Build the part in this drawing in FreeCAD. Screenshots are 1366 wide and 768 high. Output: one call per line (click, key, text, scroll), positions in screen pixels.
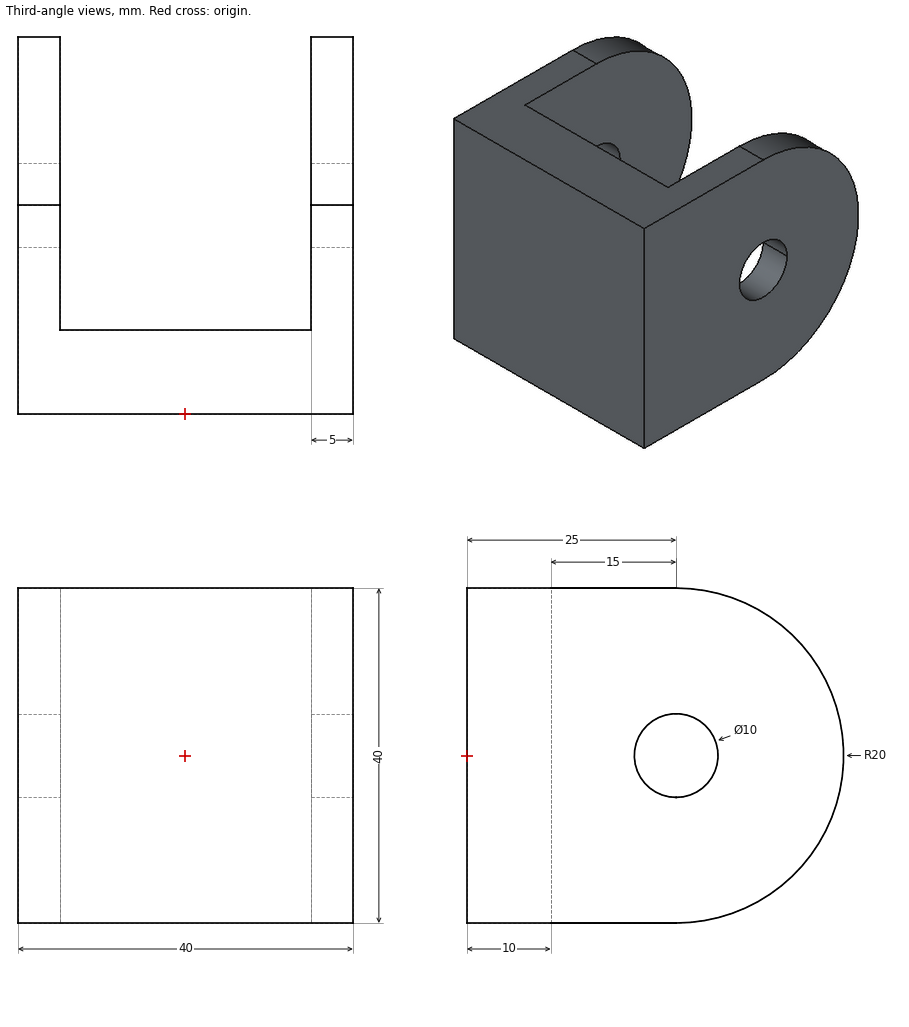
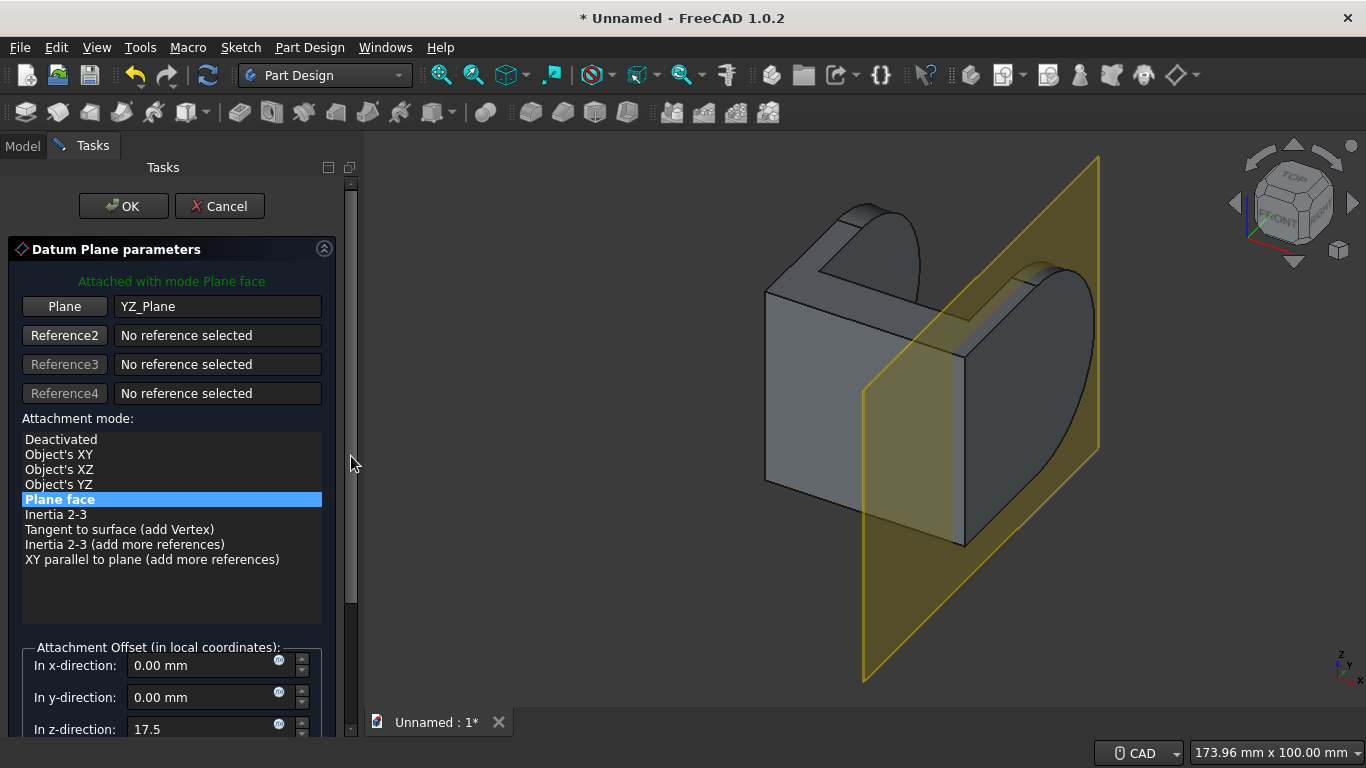
click(124, 206)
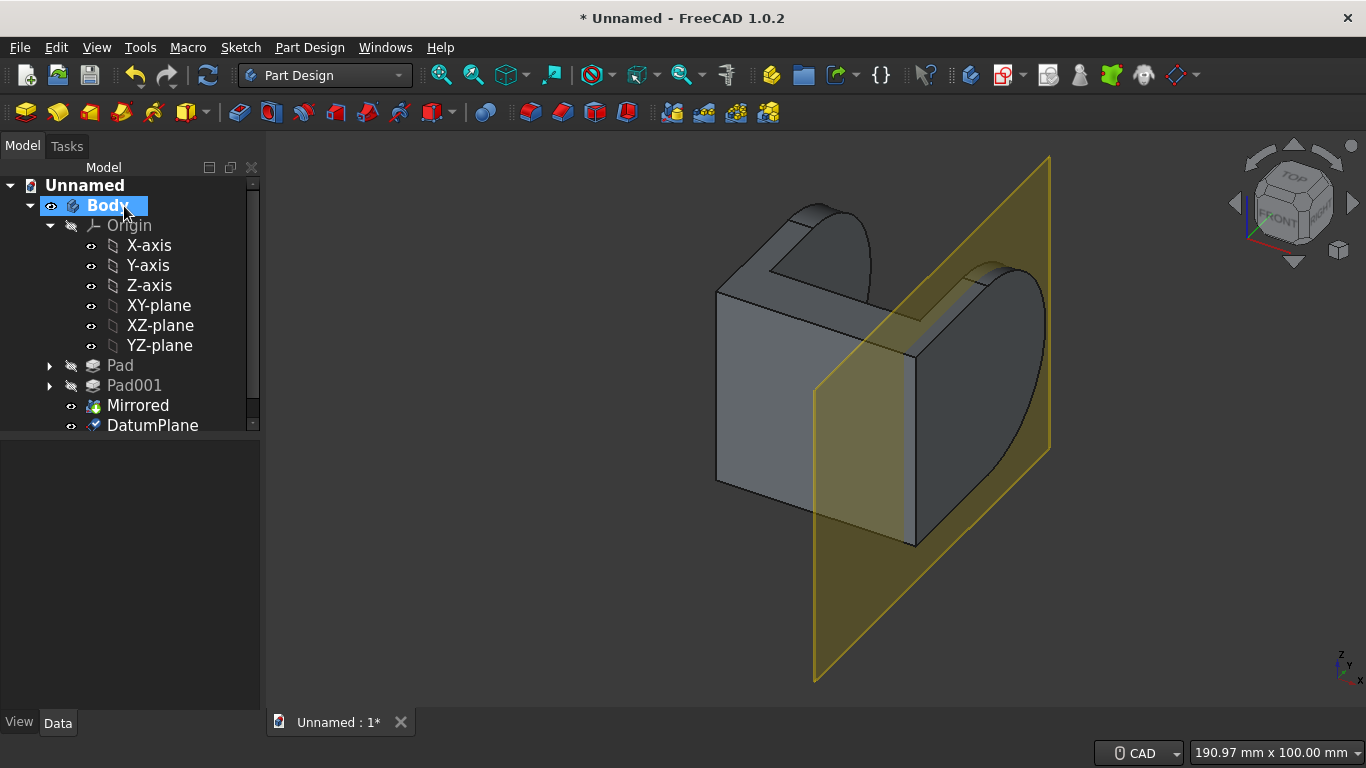
click(116, 426)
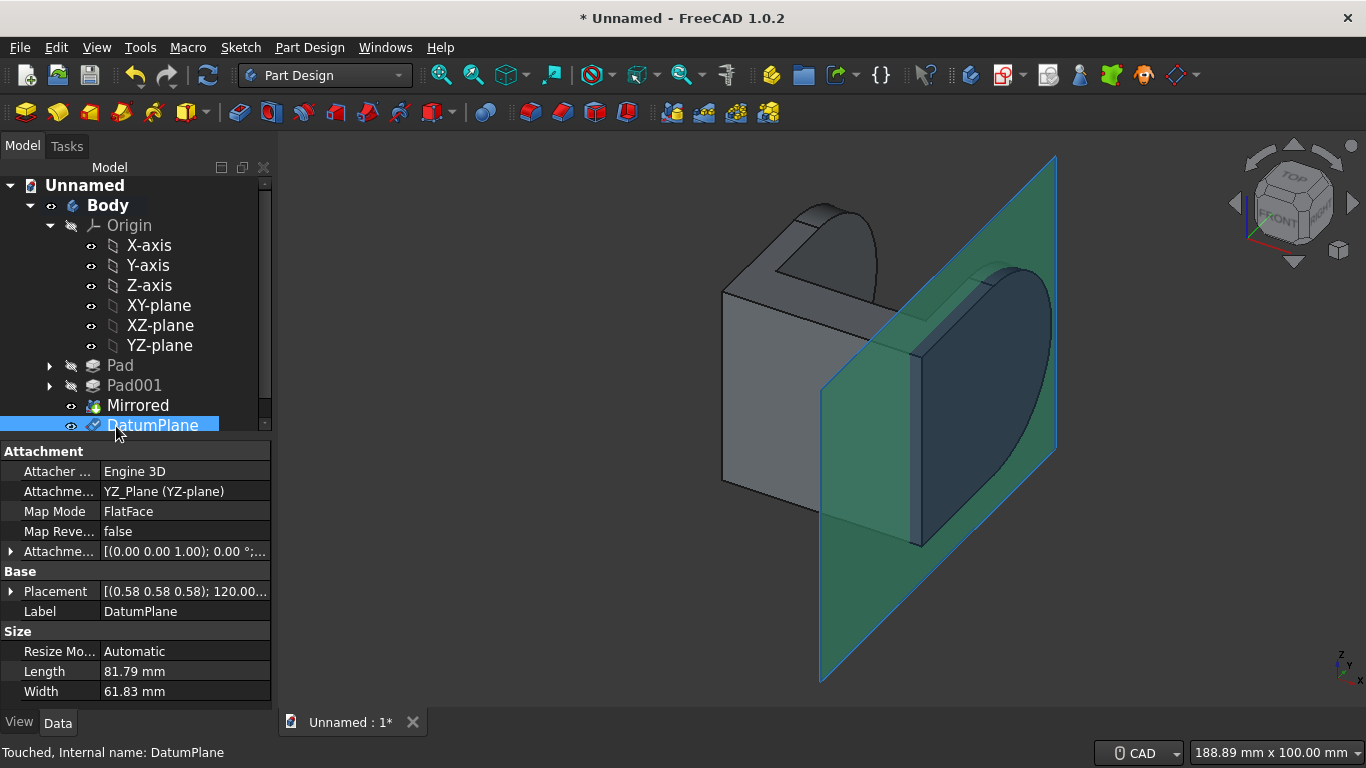
click(1004, 76)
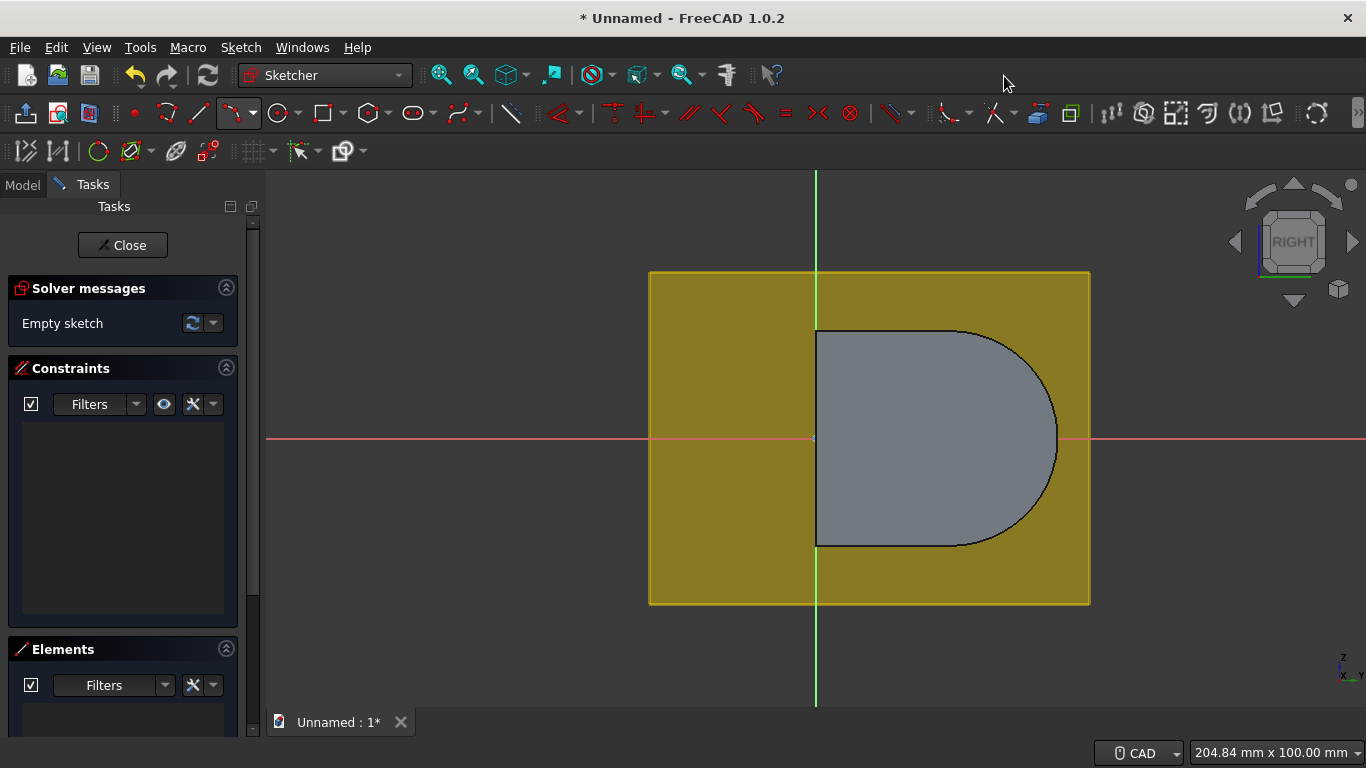
key(q)
key(s)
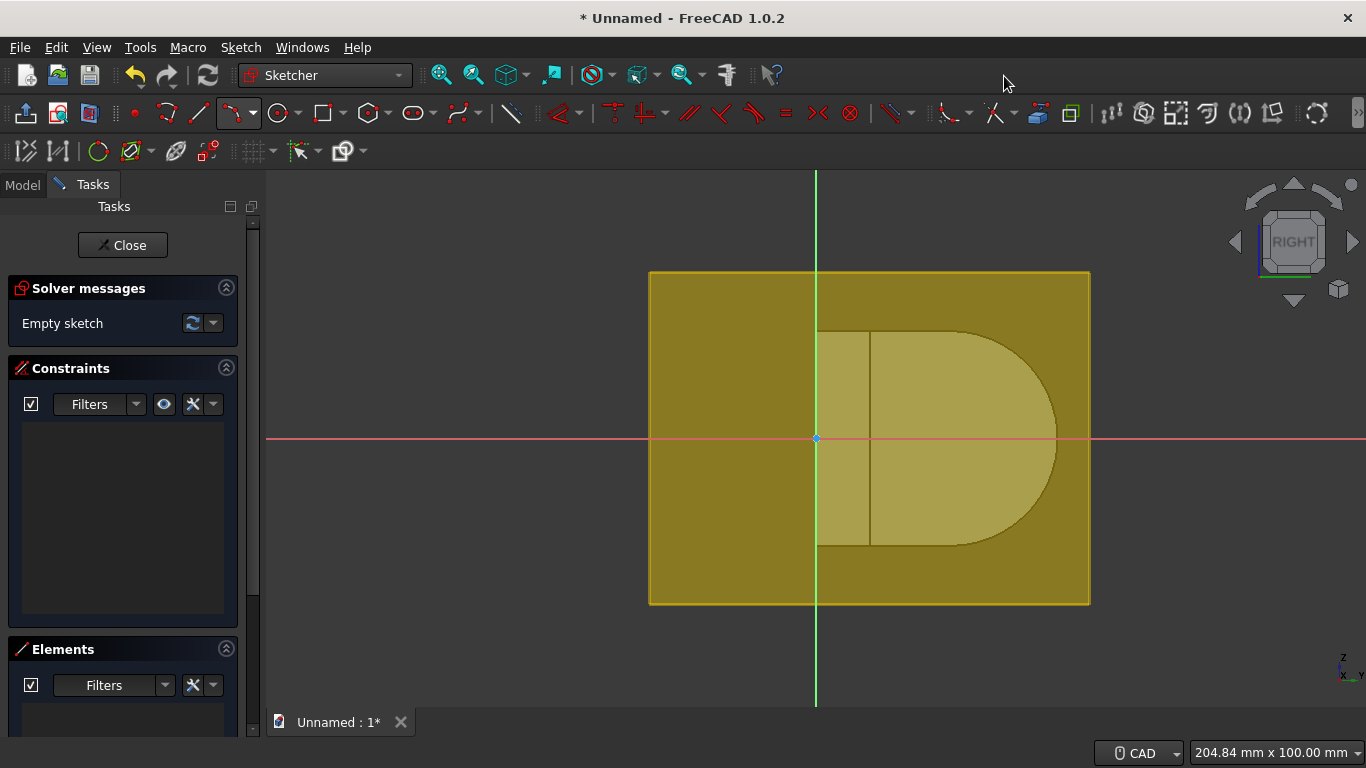
scroll(990, 438, up, 9)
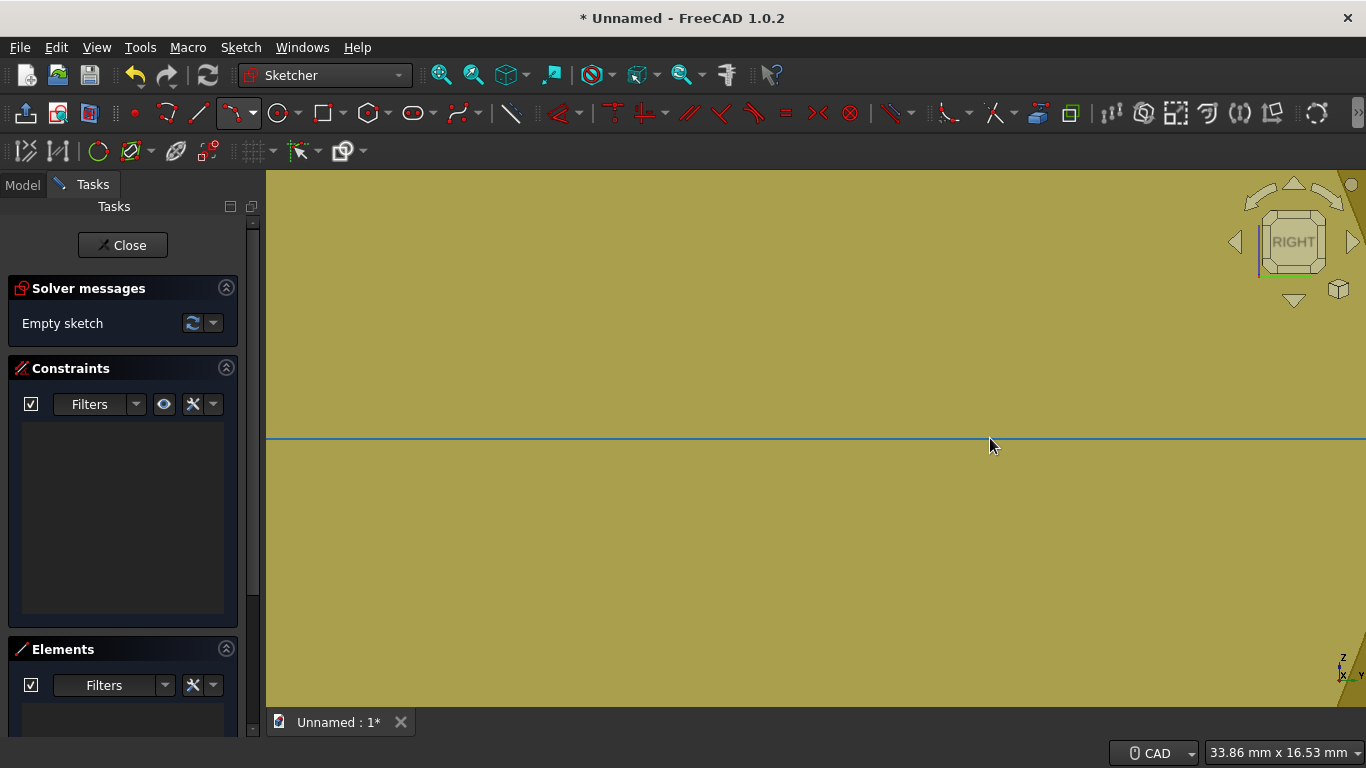
click(278, 114)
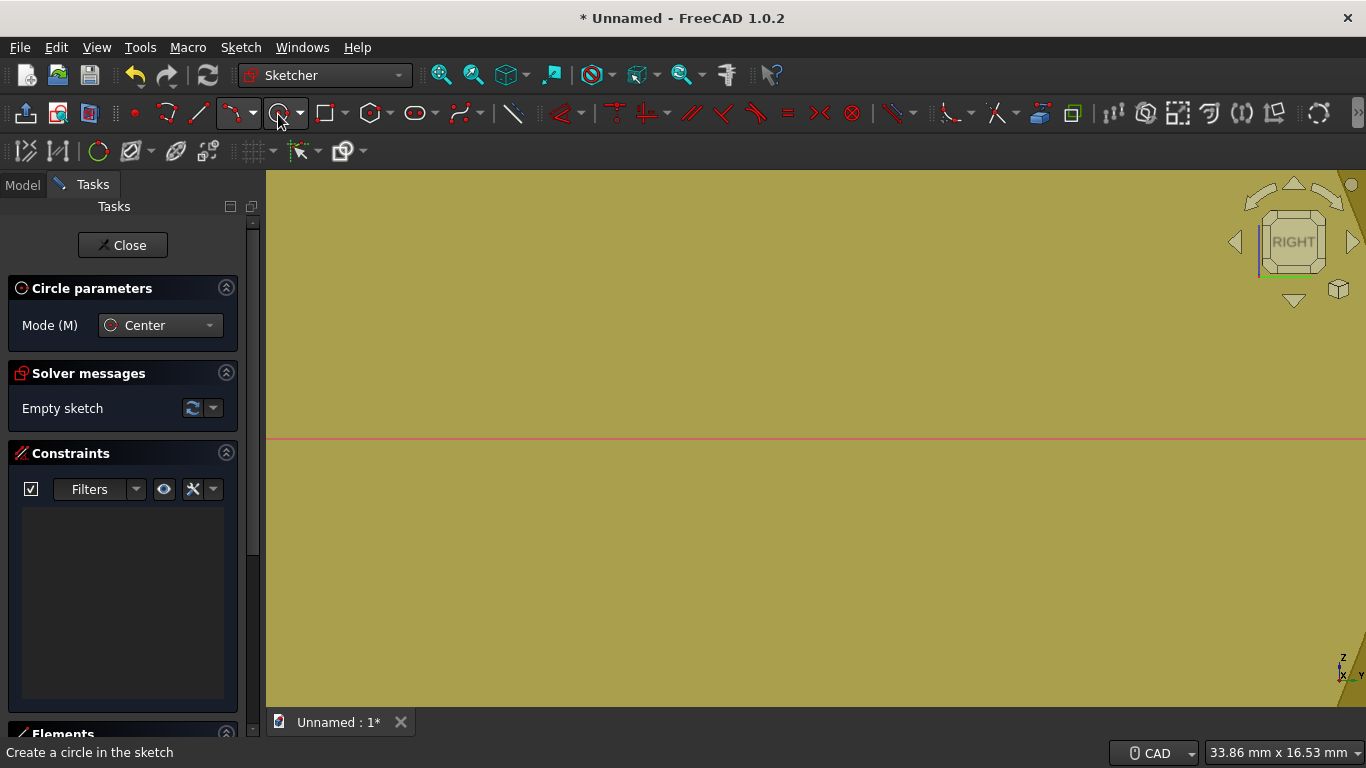
click(746, 438)
click(861, 324)
key(Escape)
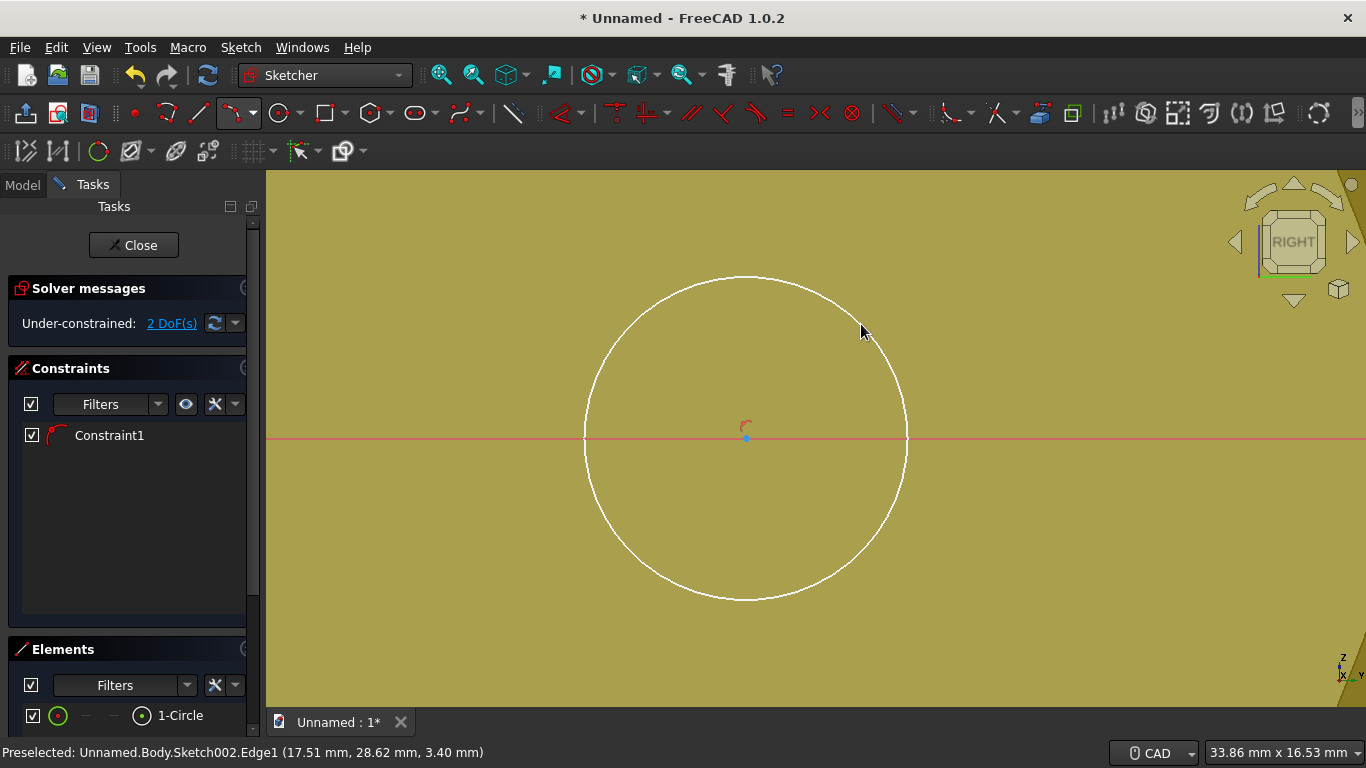
click(560, 114)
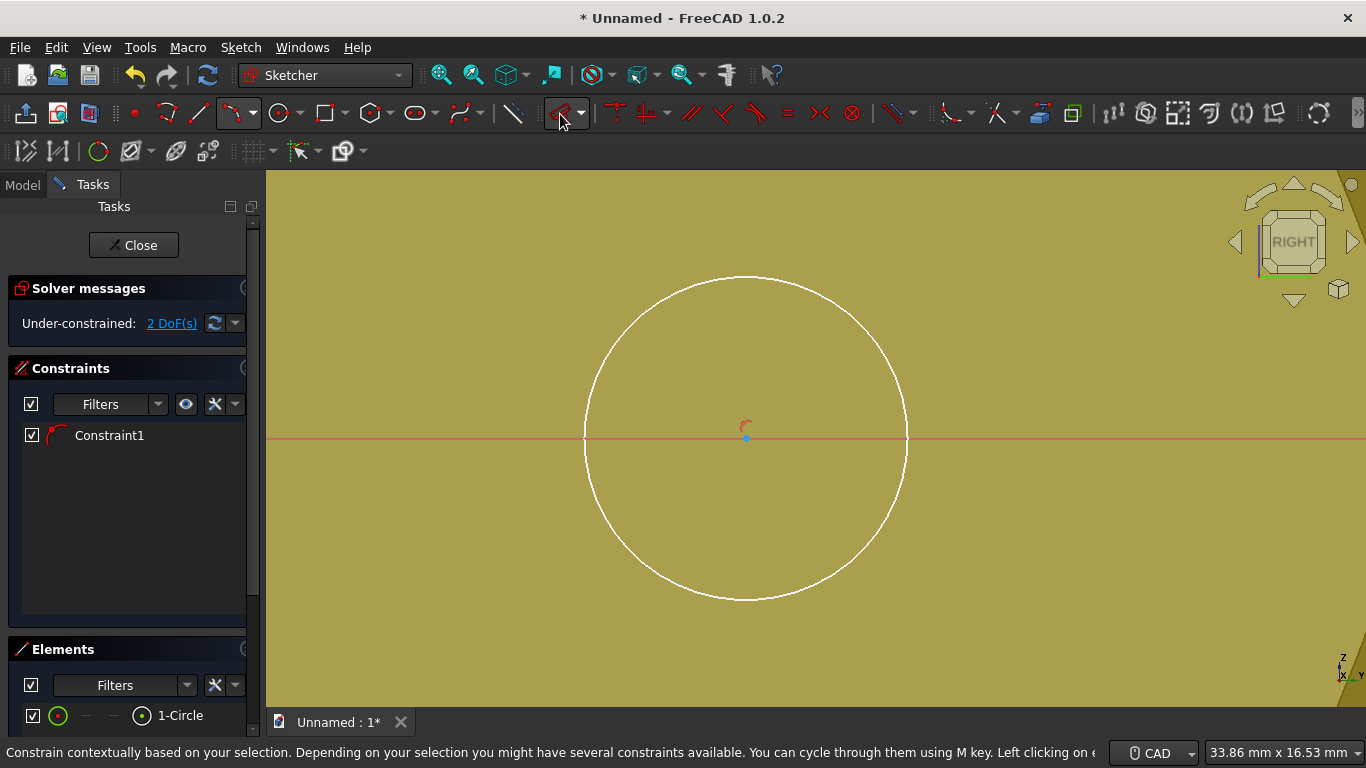
click(860, 324)
click(883, 301)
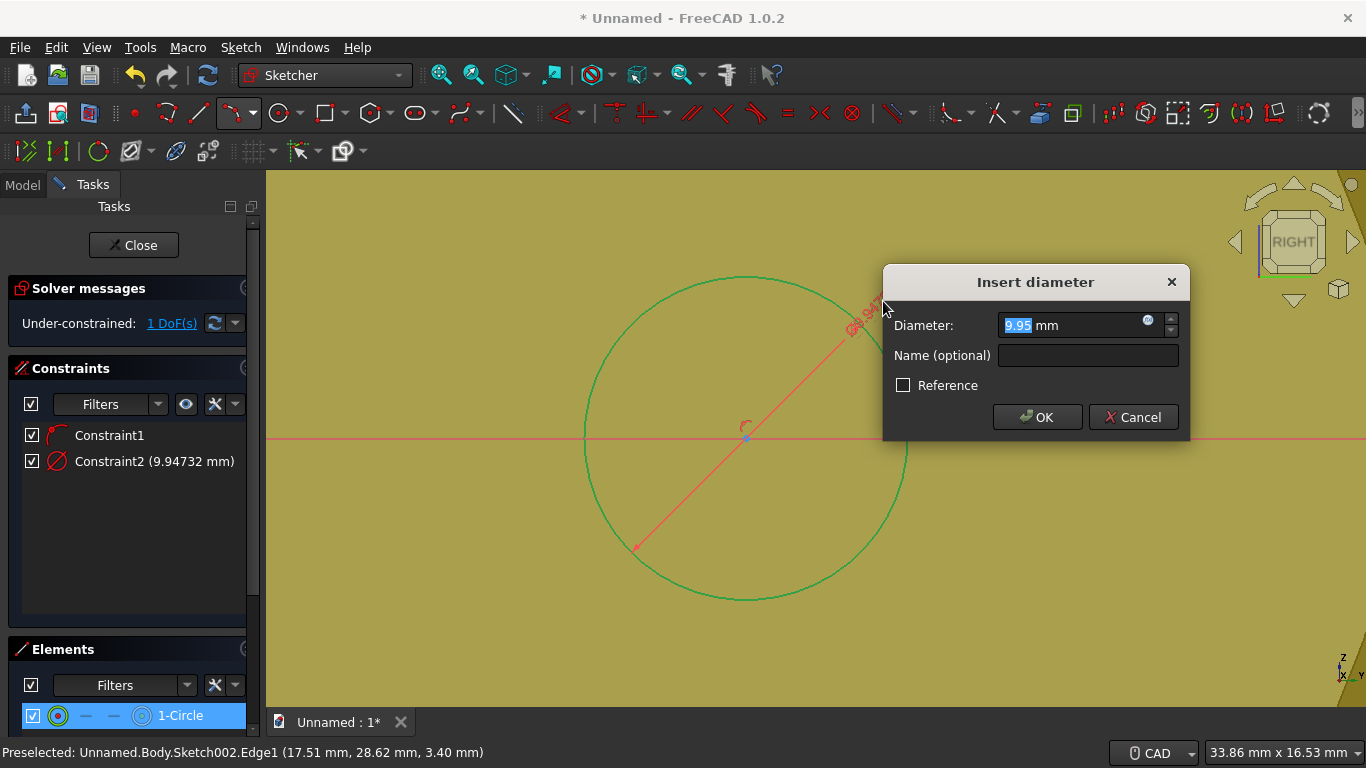
text(10)
key(Return)